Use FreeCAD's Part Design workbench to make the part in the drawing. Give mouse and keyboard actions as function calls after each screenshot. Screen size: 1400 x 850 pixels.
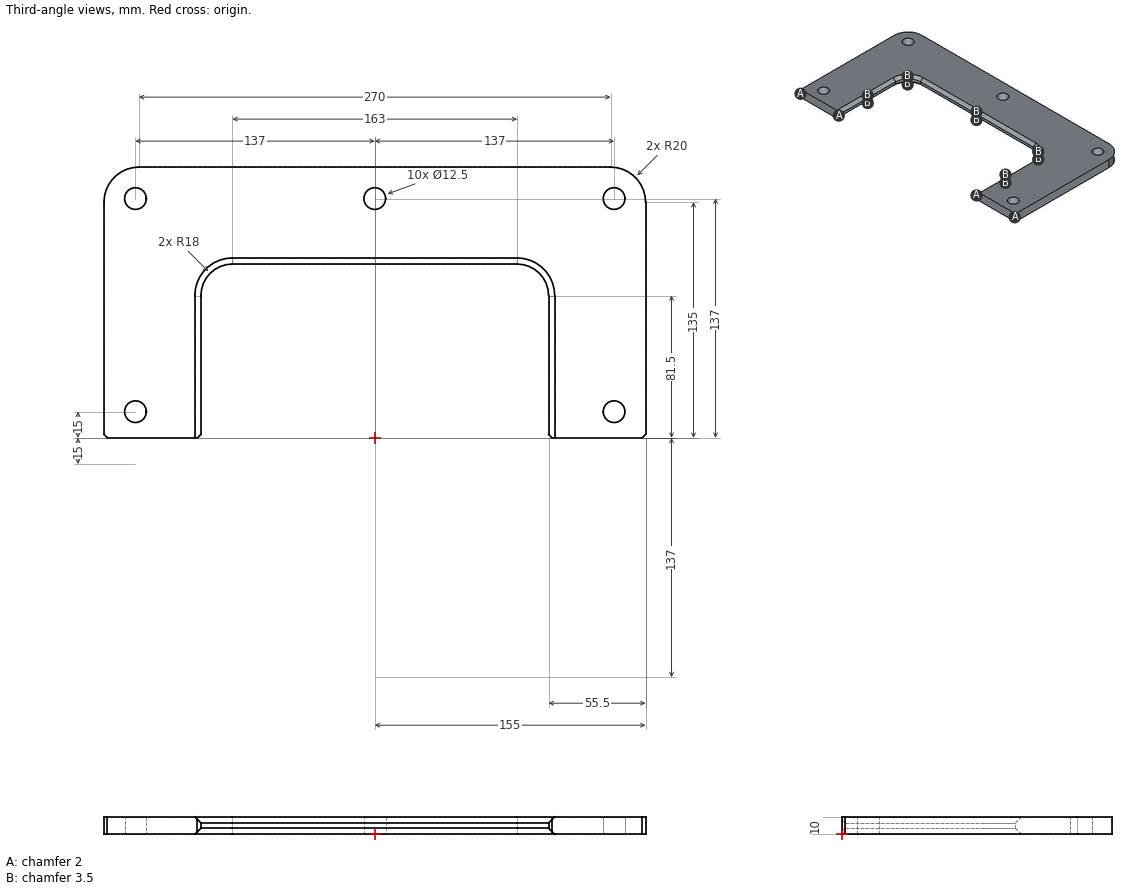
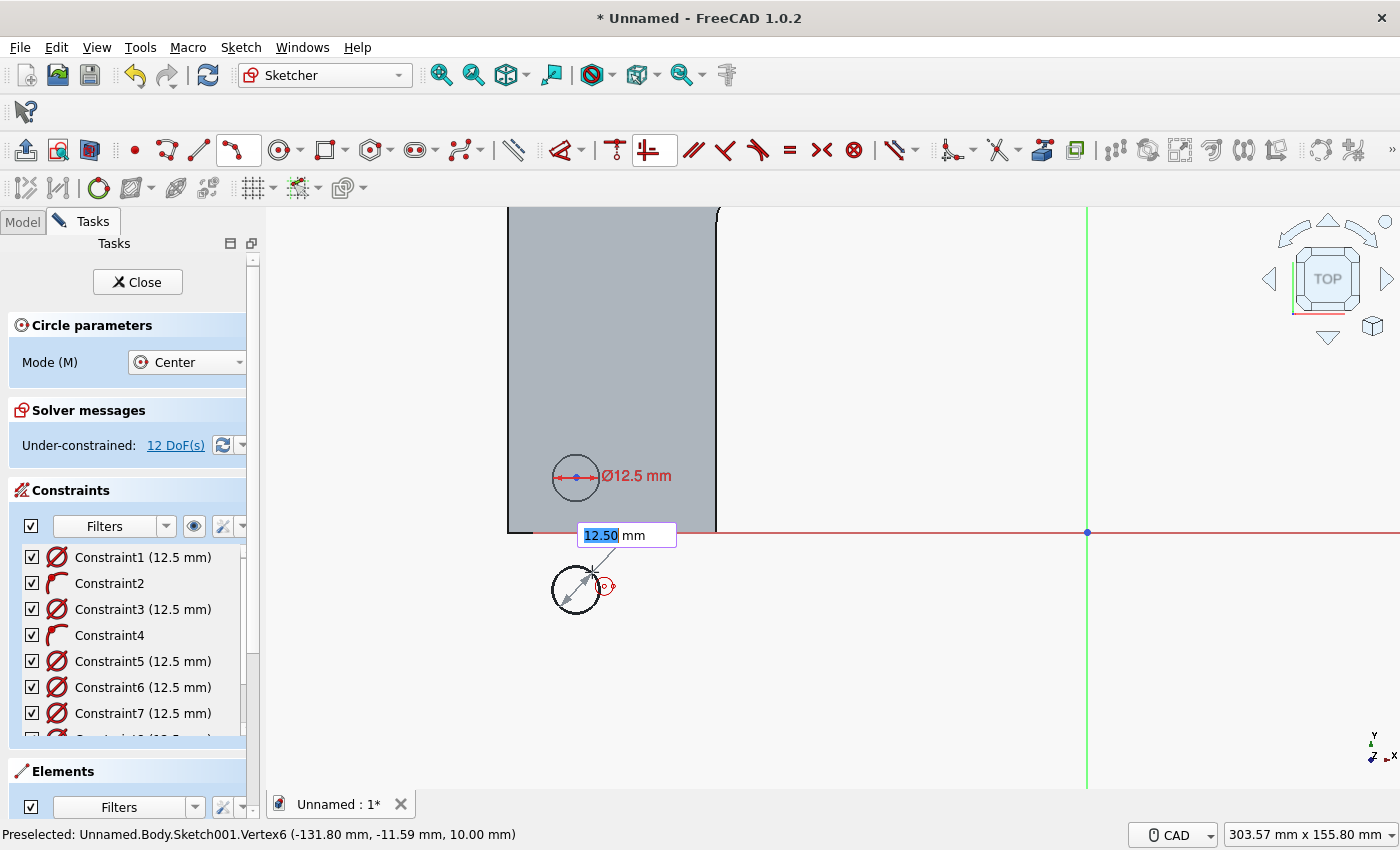
text(12.5)
key(Return)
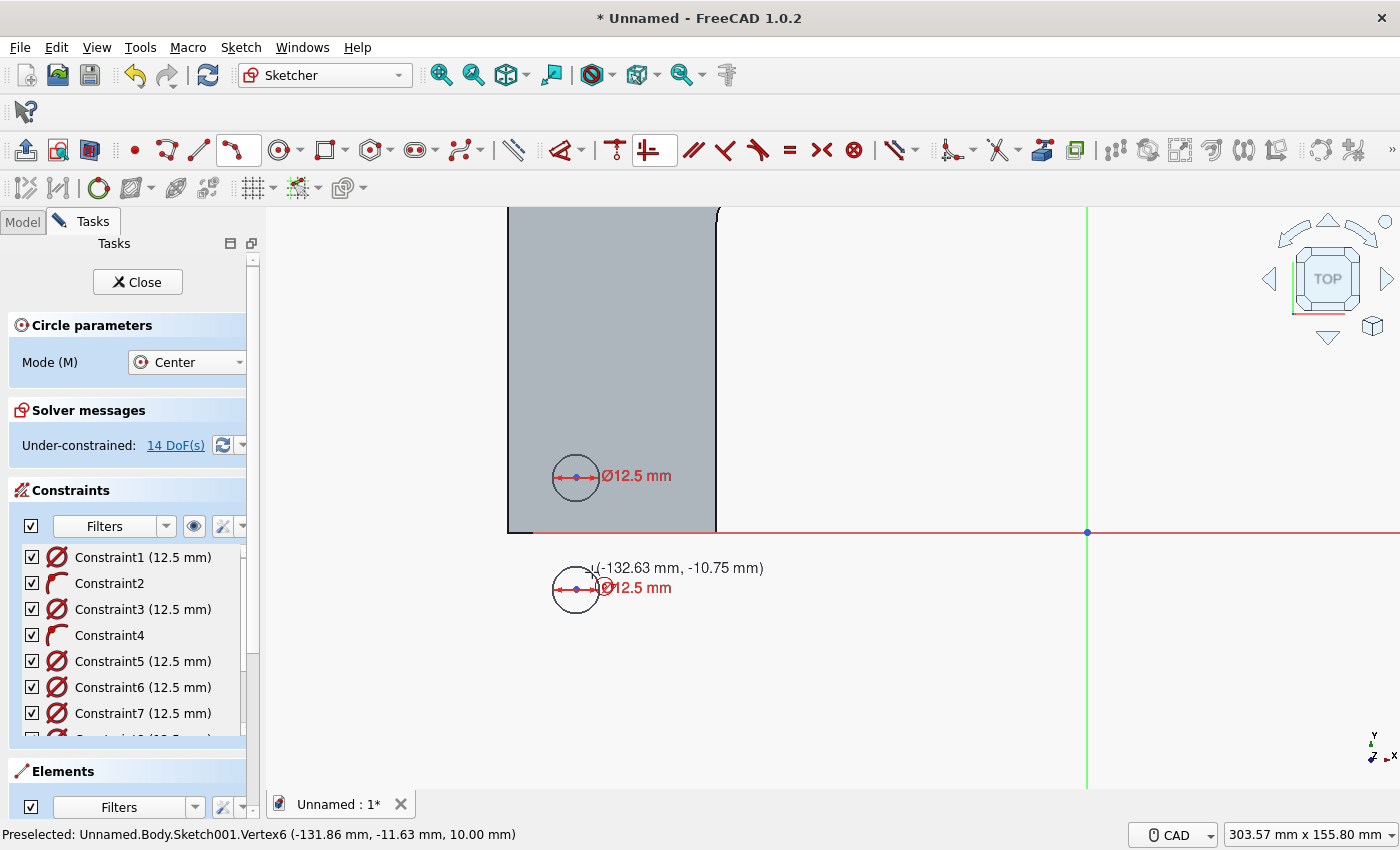
scroll(577, 478, down, 5)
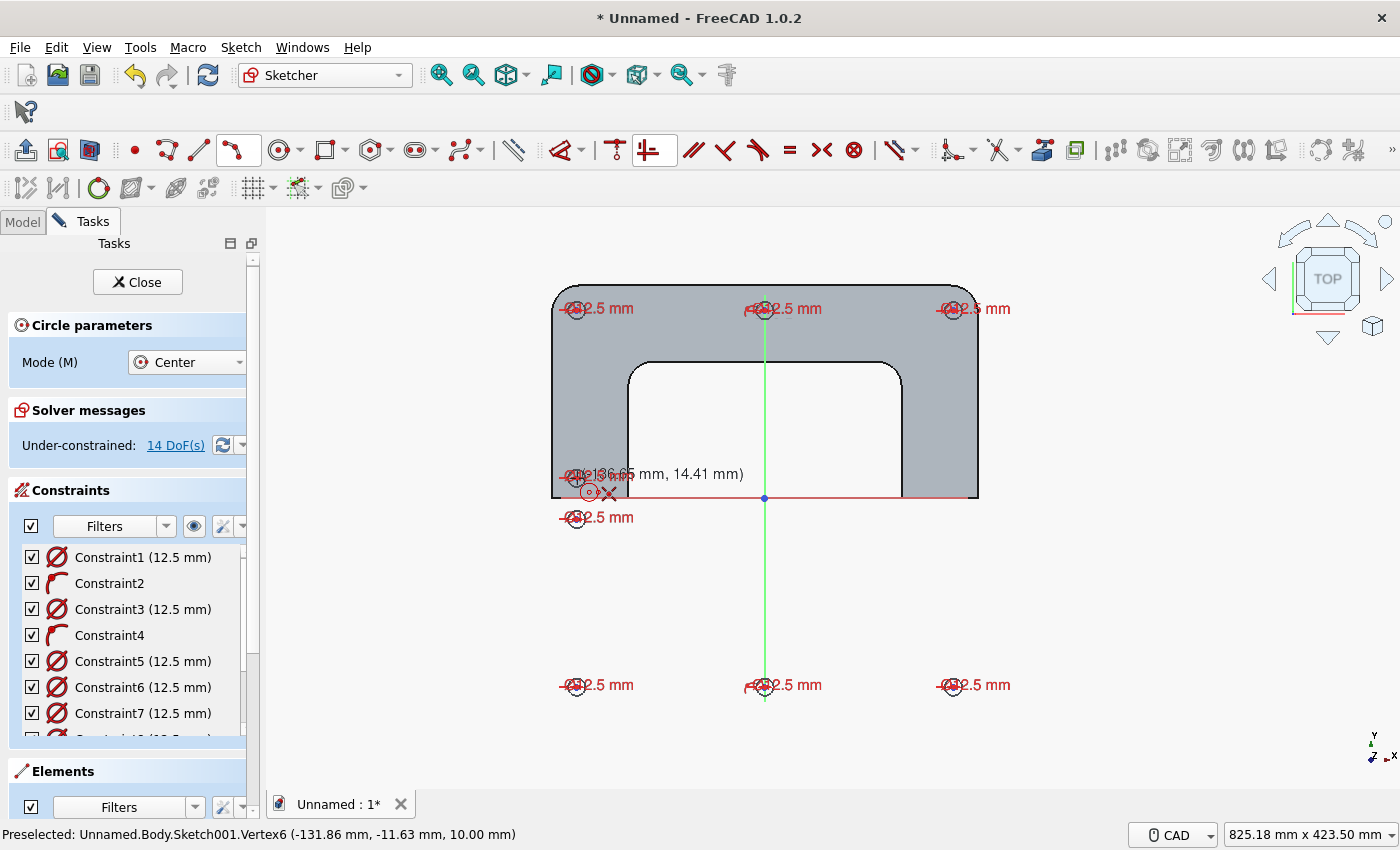
scroll(953, 519, up, 5)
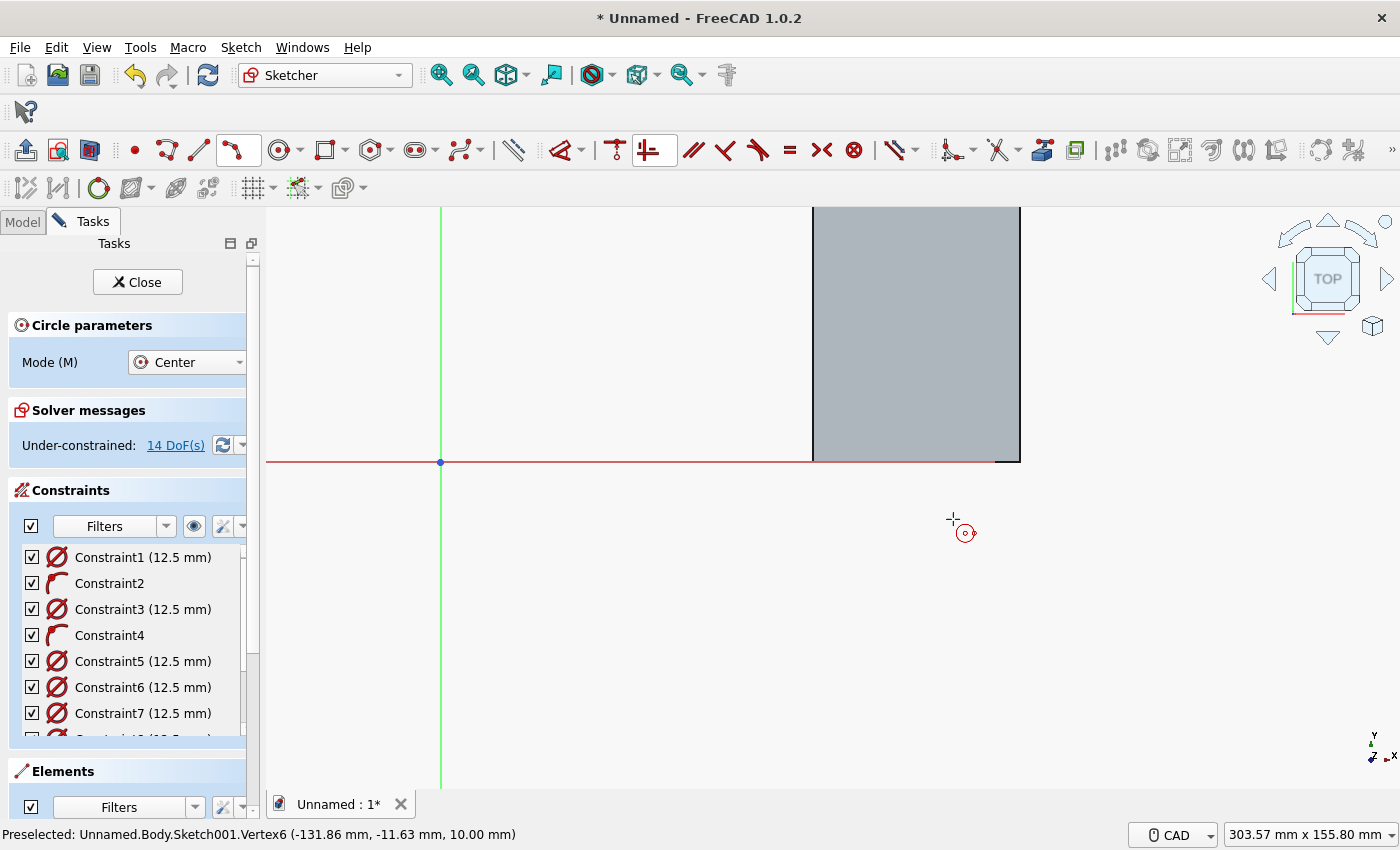
click(953, 518)
move(969, 502)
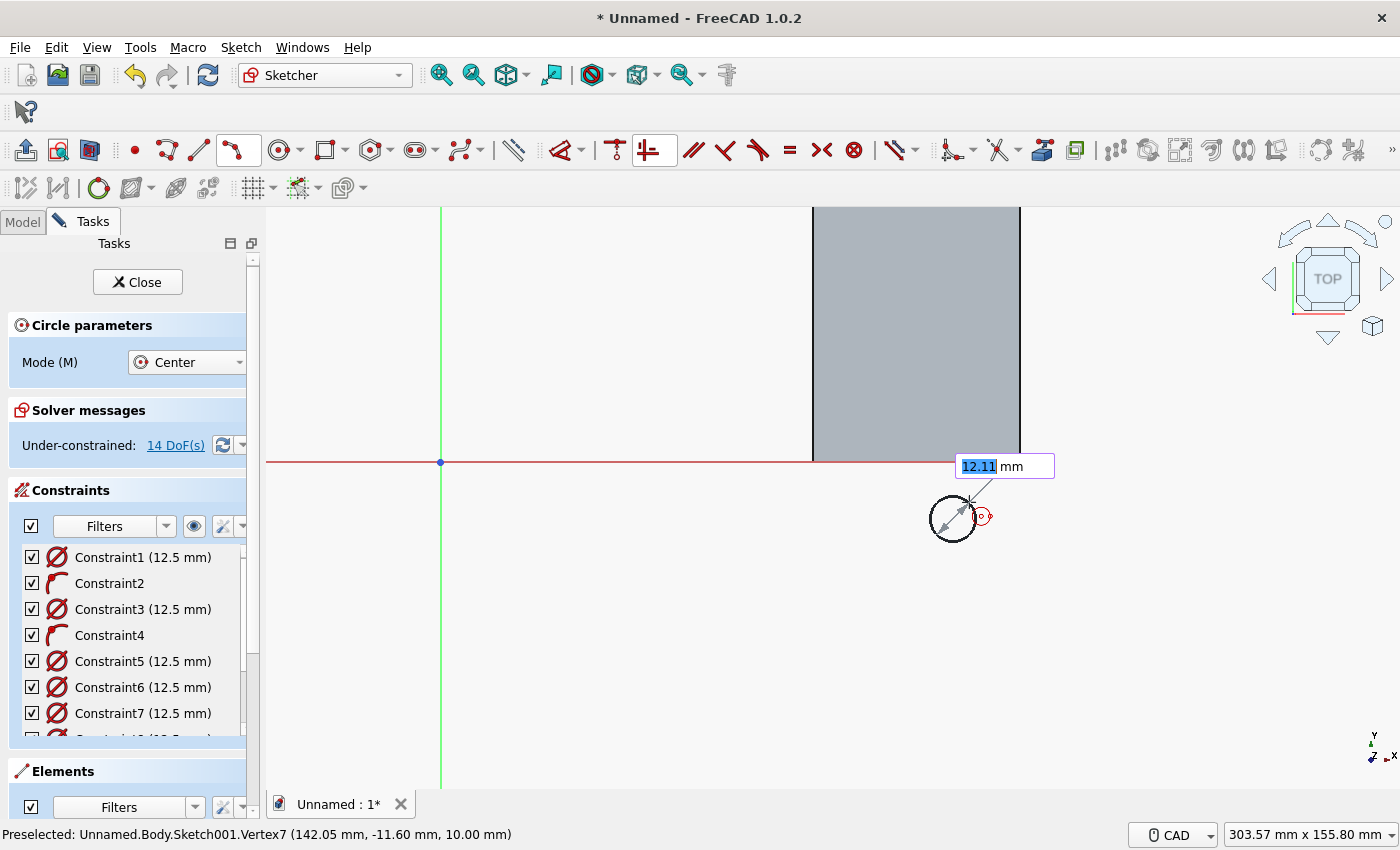
text(12.5)
key(Return)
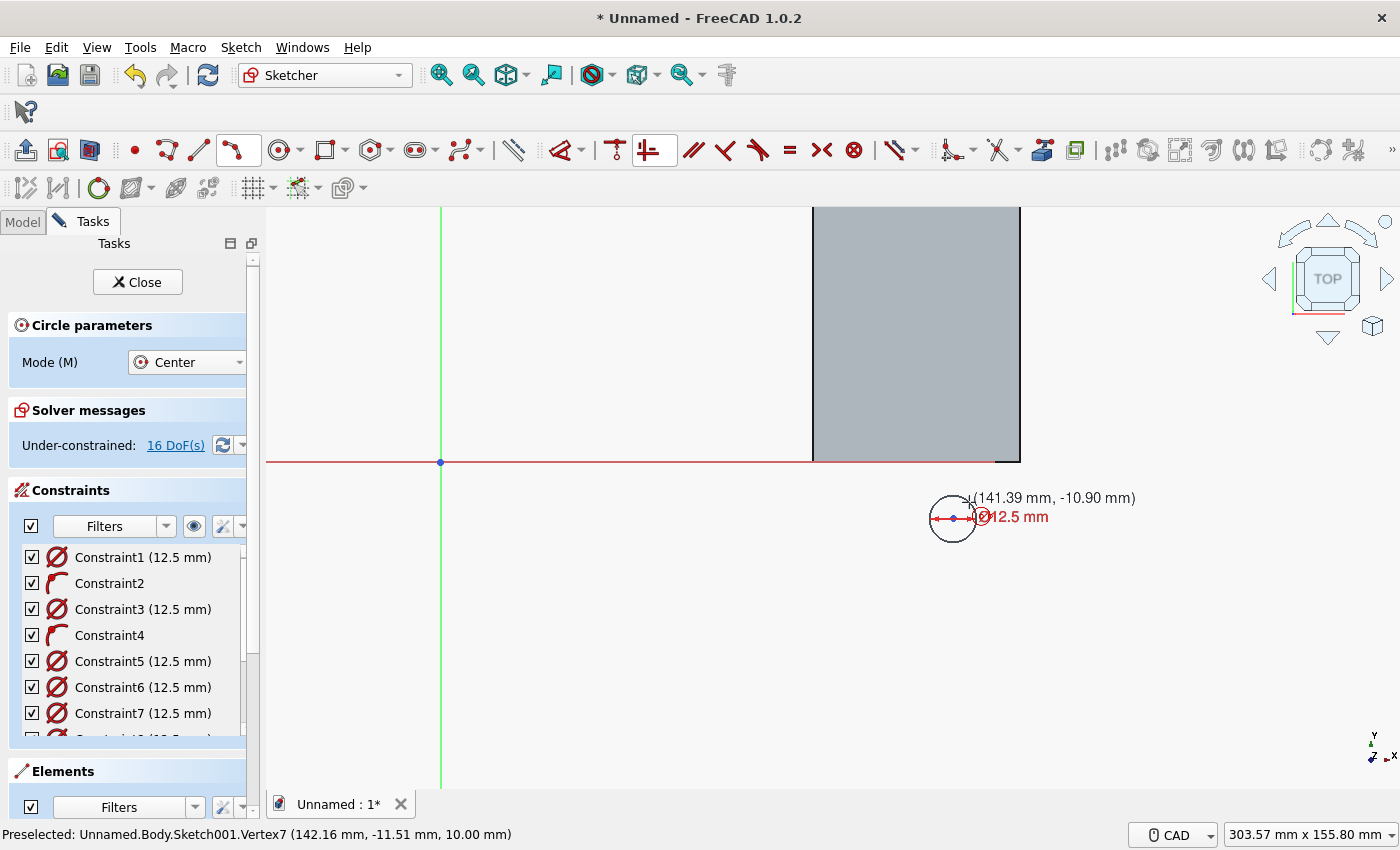
click(953, 406)
move(969, 390)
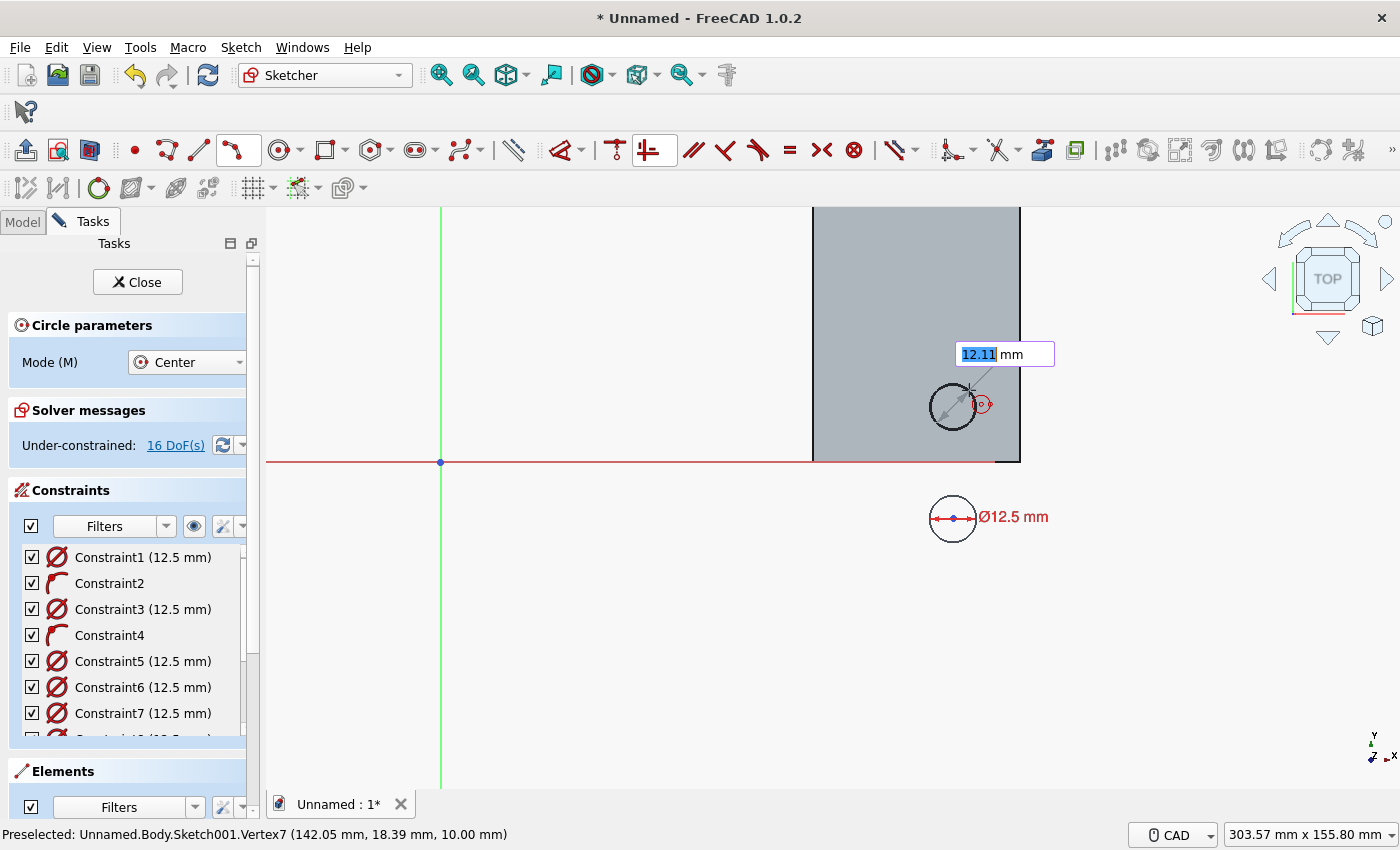
text(12.5)
key(Return)
key(Escape)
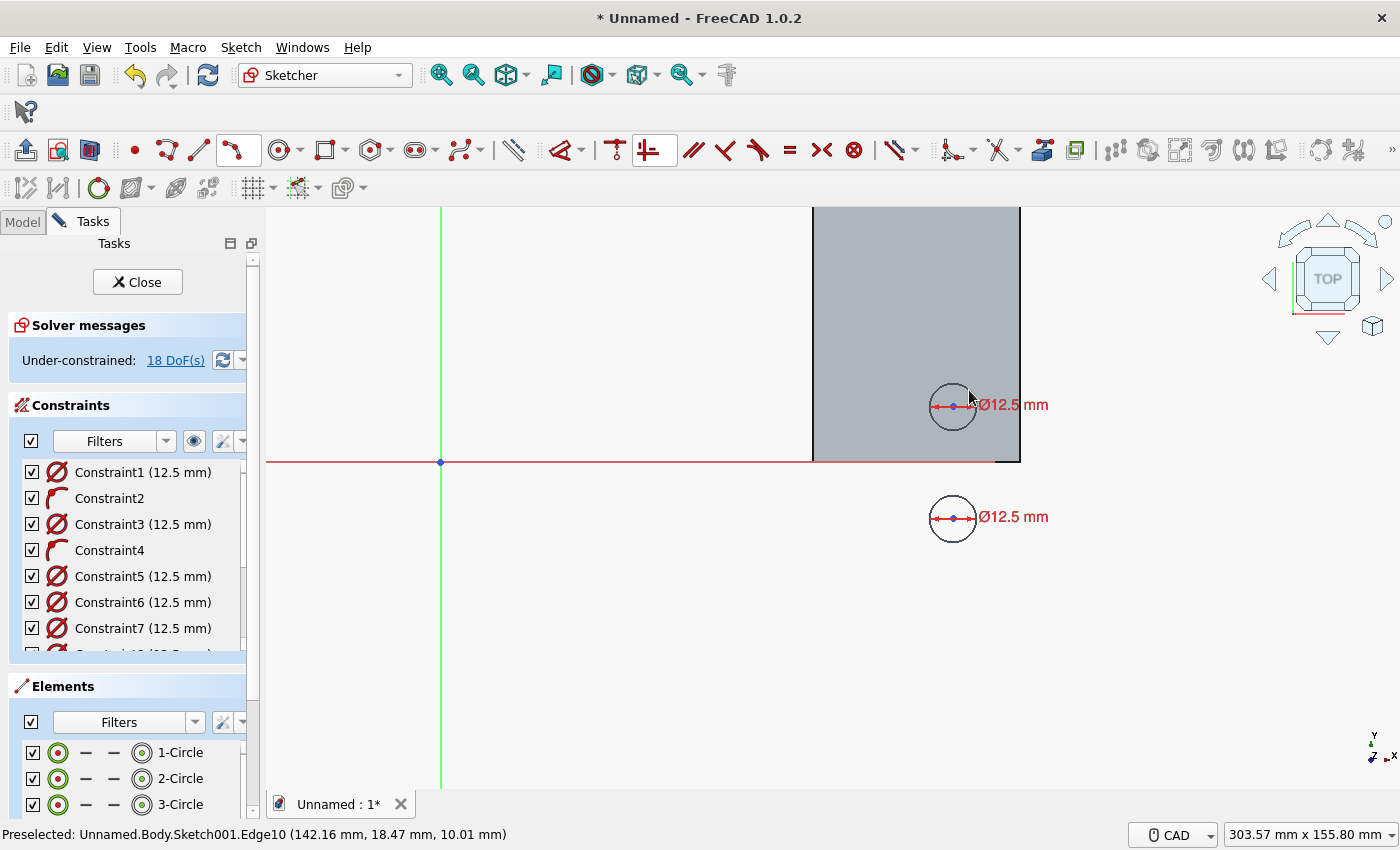
scroll(953, 519, down, 5)